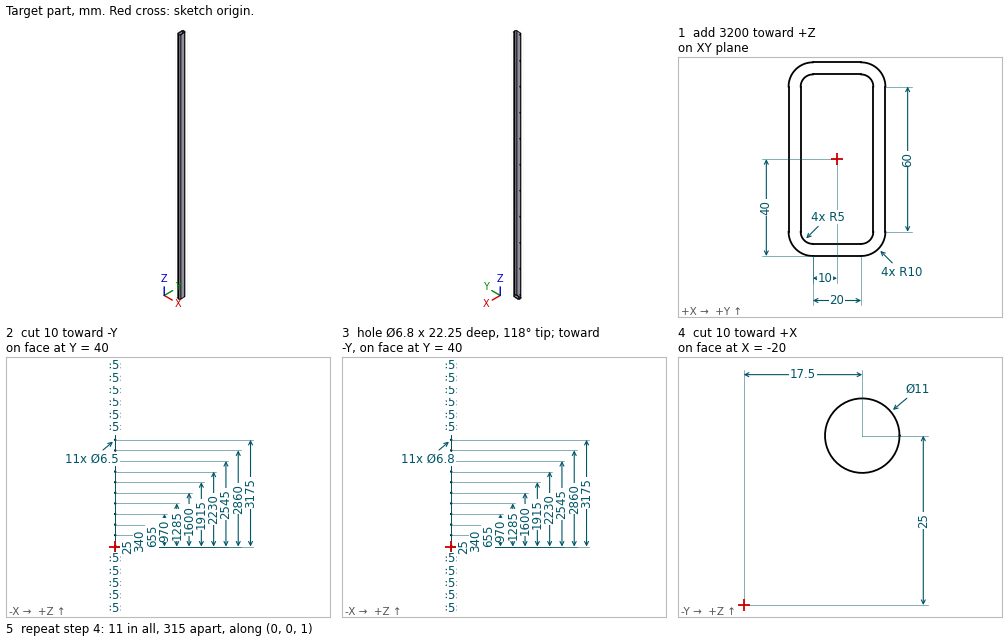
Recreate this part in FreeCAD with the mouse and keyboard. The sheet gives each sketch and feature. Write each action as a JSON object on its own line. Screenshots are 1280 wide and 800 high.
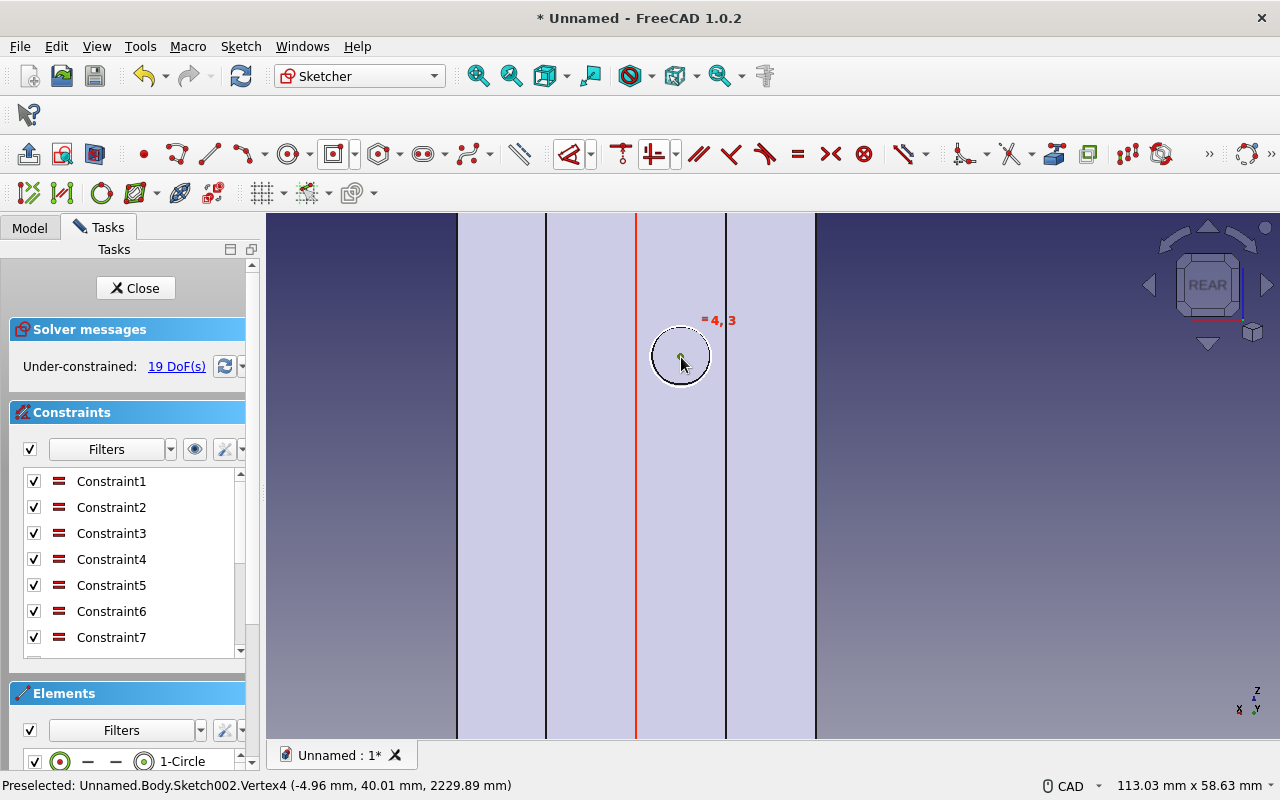
{"action": "left_click", "coordinate": [590, 154]}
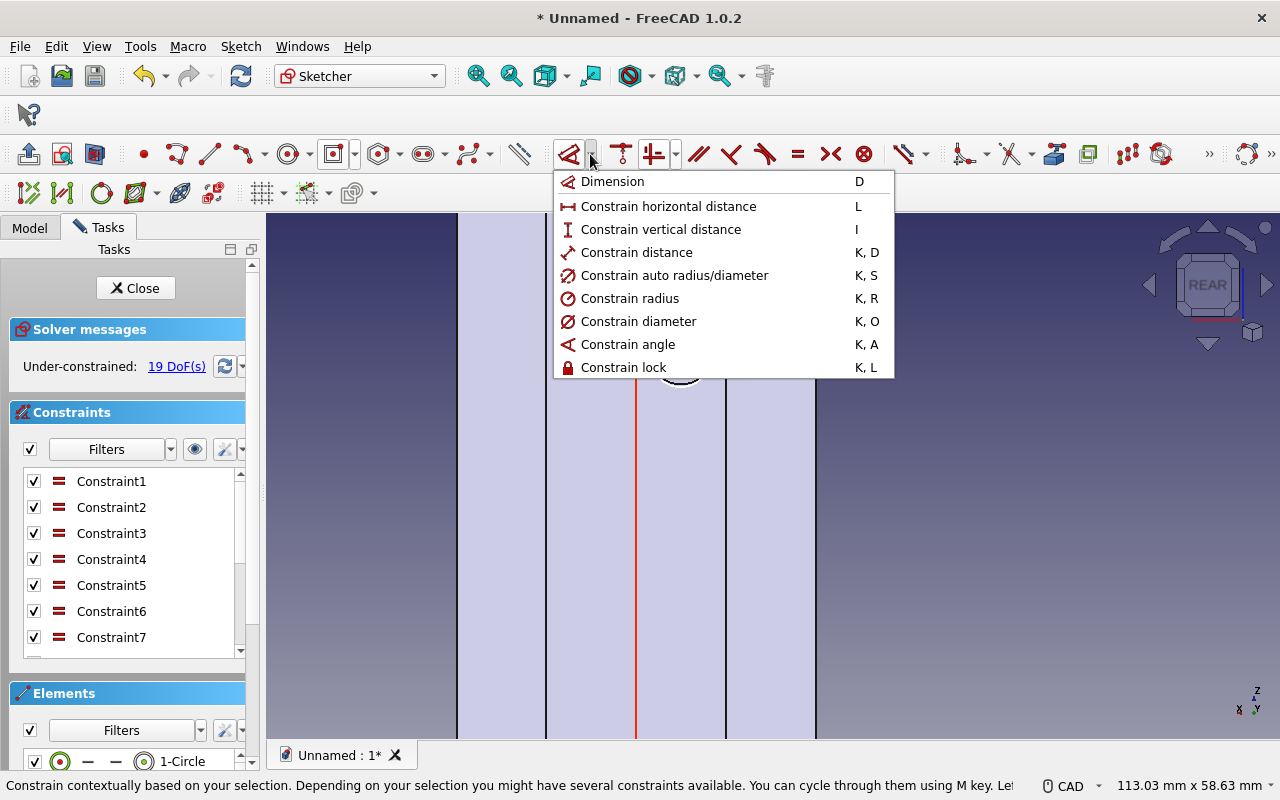
{"action": "left_click", "coordinate": [724, 206]}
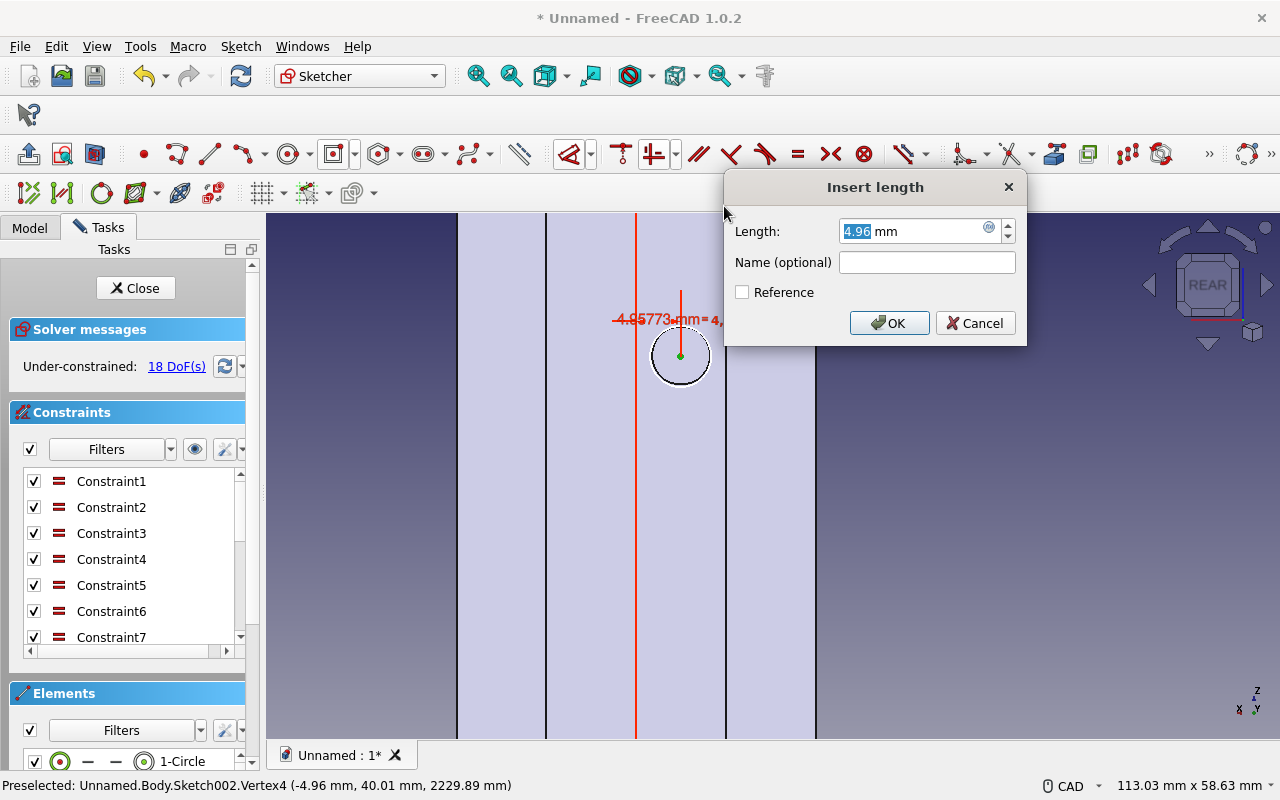
{"action": "type", "text": "5"}
{"action": "key", "text": "Return"}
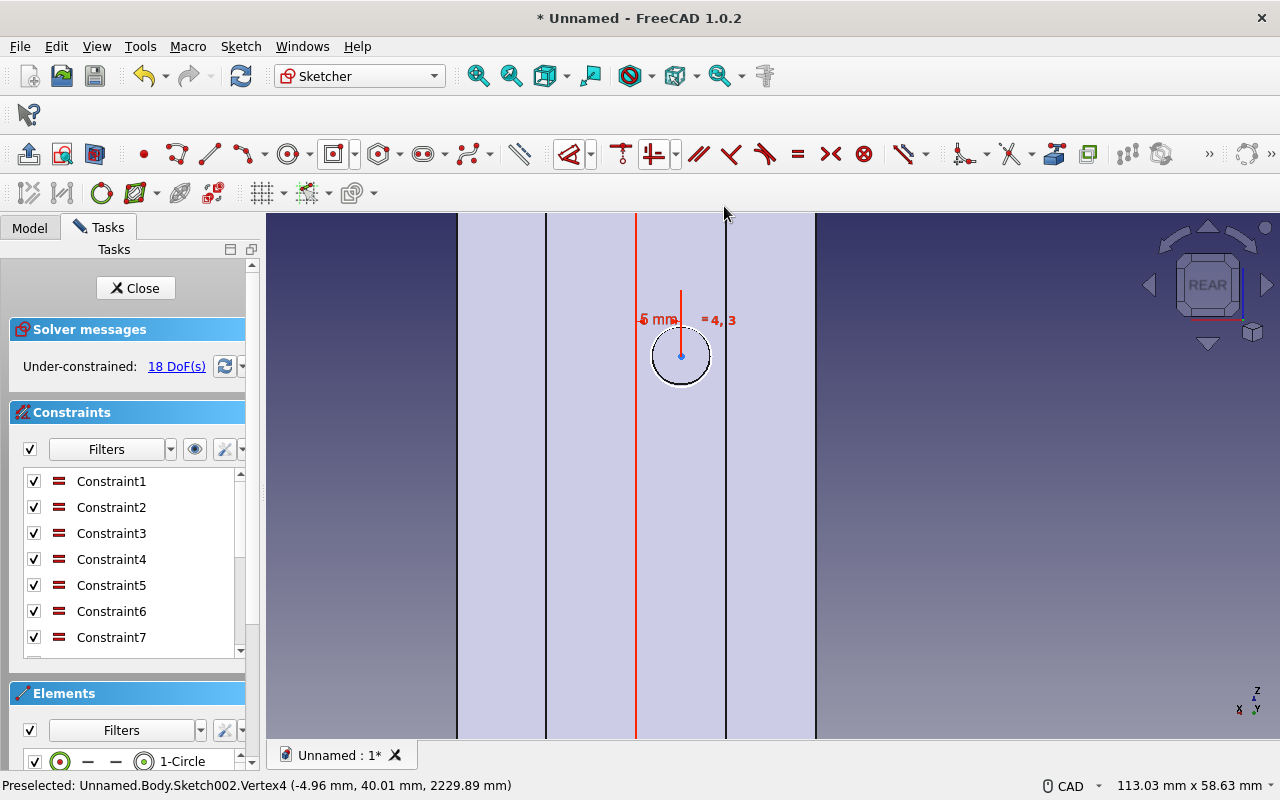
{"action": "scroll", "coordinate": [704, 476], "scroll_direction": "down", "scroll_amount": 15}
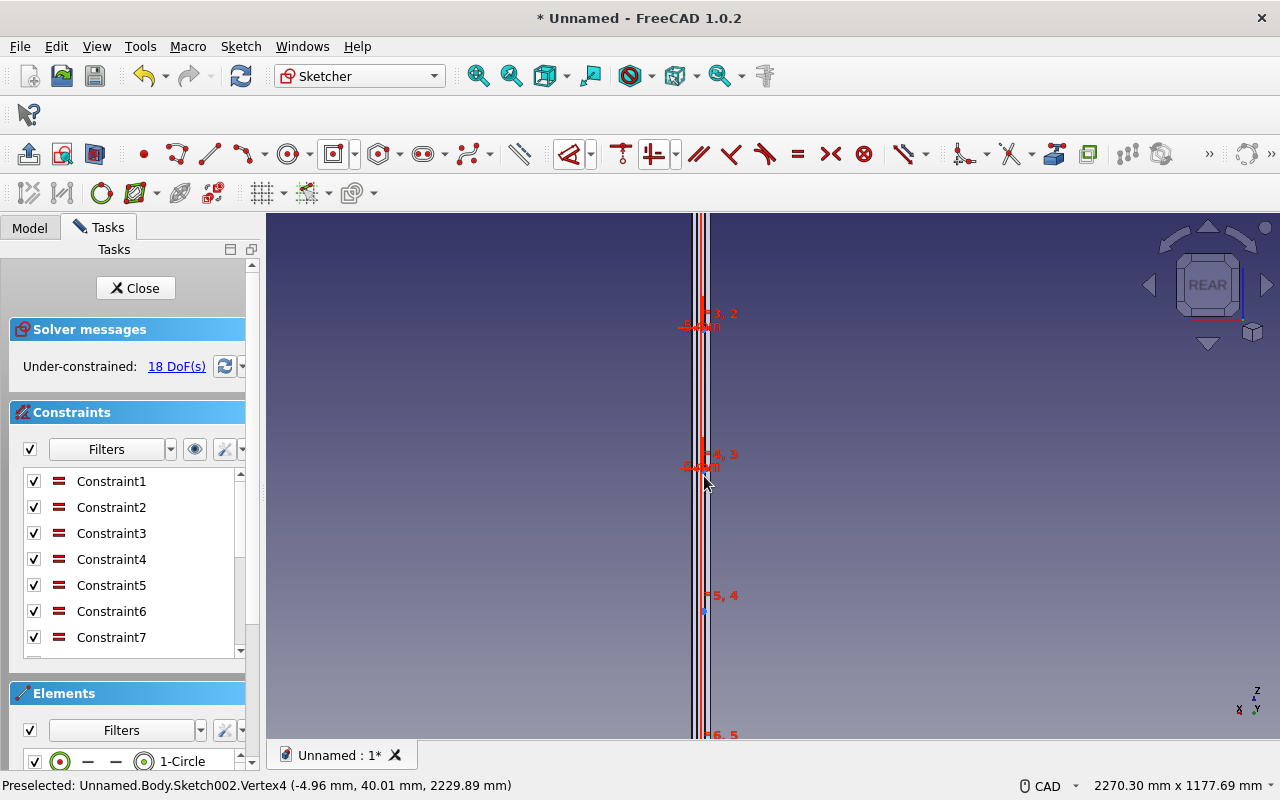
{"action": "scroll", "coordinate": [705, 384], "scroll_direction": "down", "scroll_amount": 7}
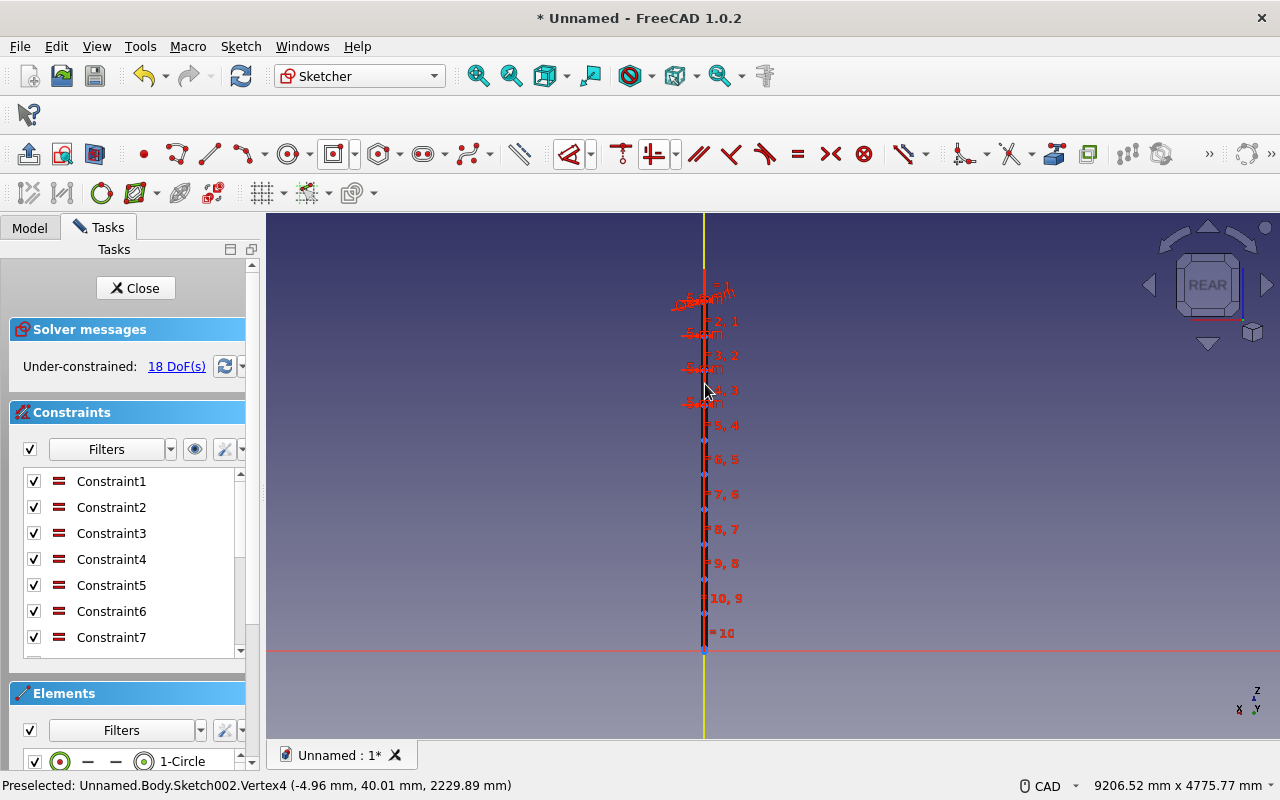
{"action": "scroll", "coordinate": [705, 440], "scroll_direction": "up", "scroll_amount": 22}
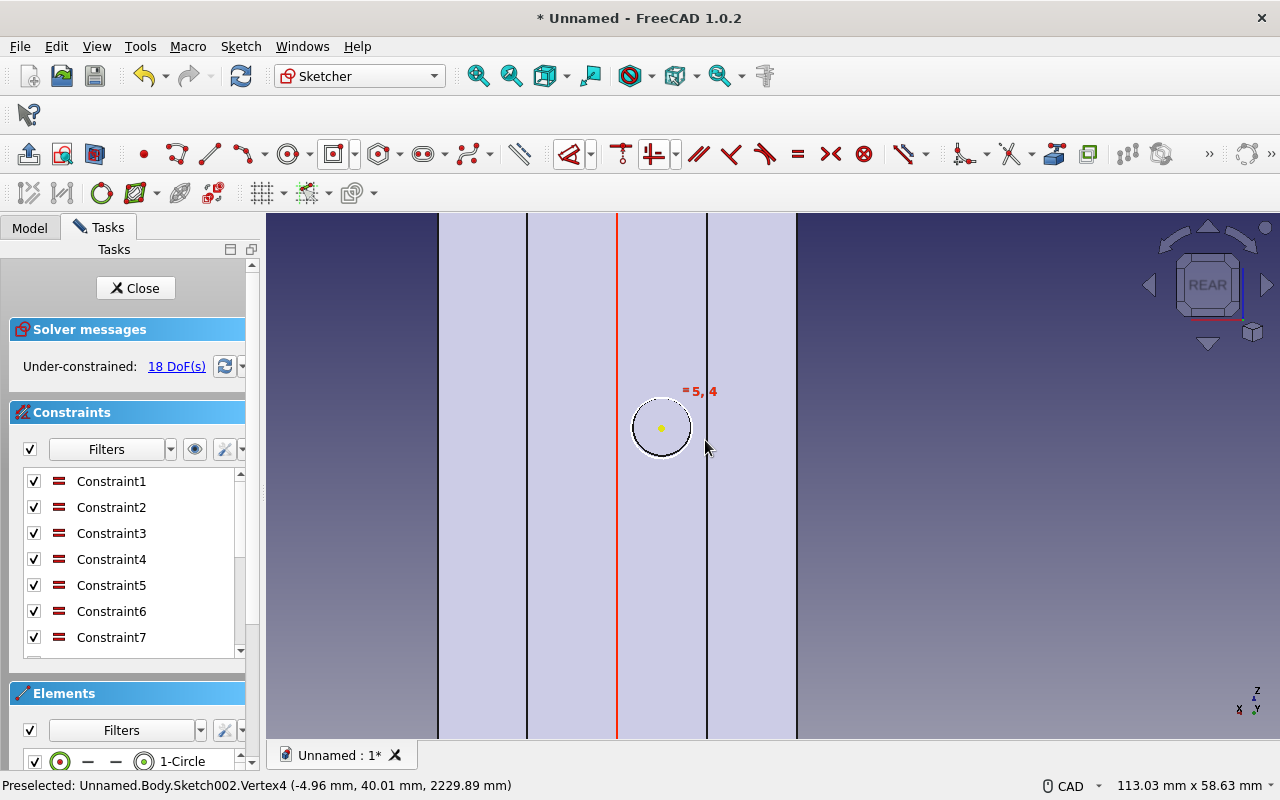
{"action": "left_click", "coordinate": [662, 428]}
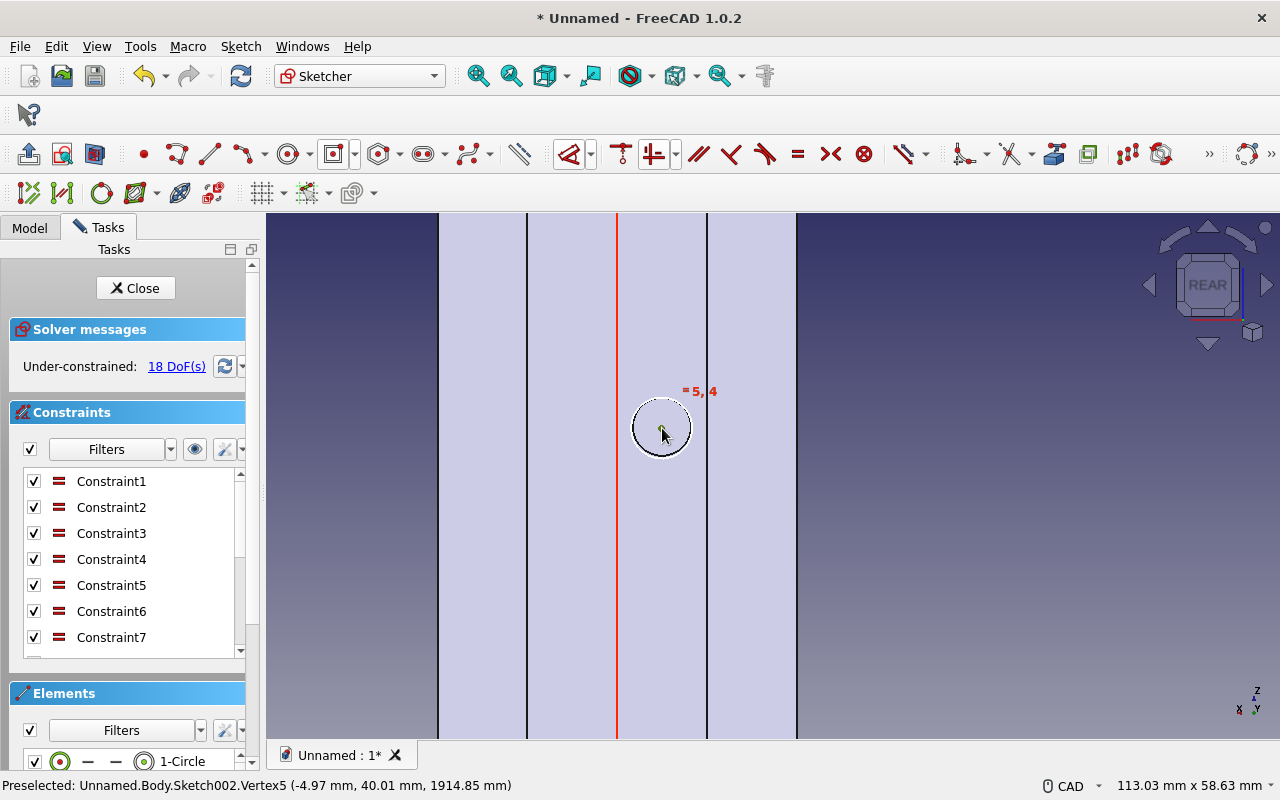
{"action": "key", "text": "l"}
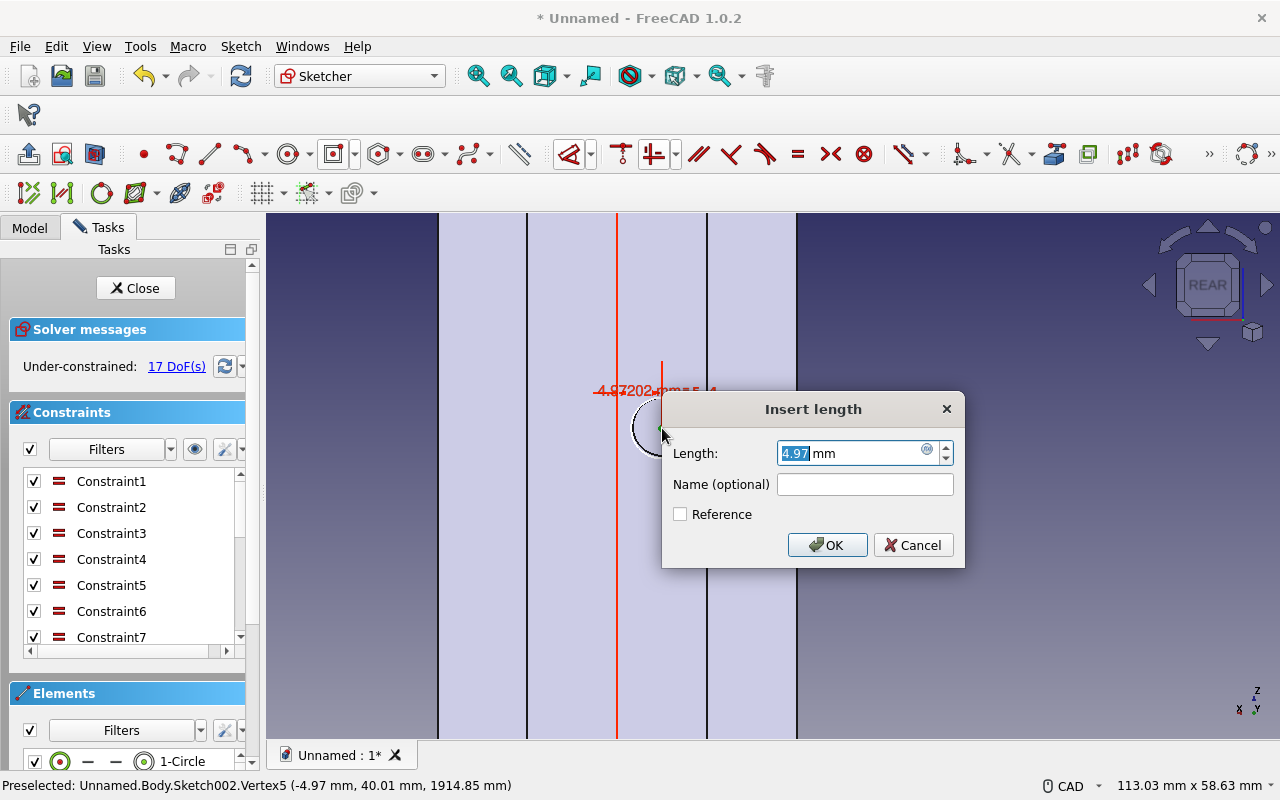
{"action": "type", "text": "5"}
{"action": "key", "text": "Return"}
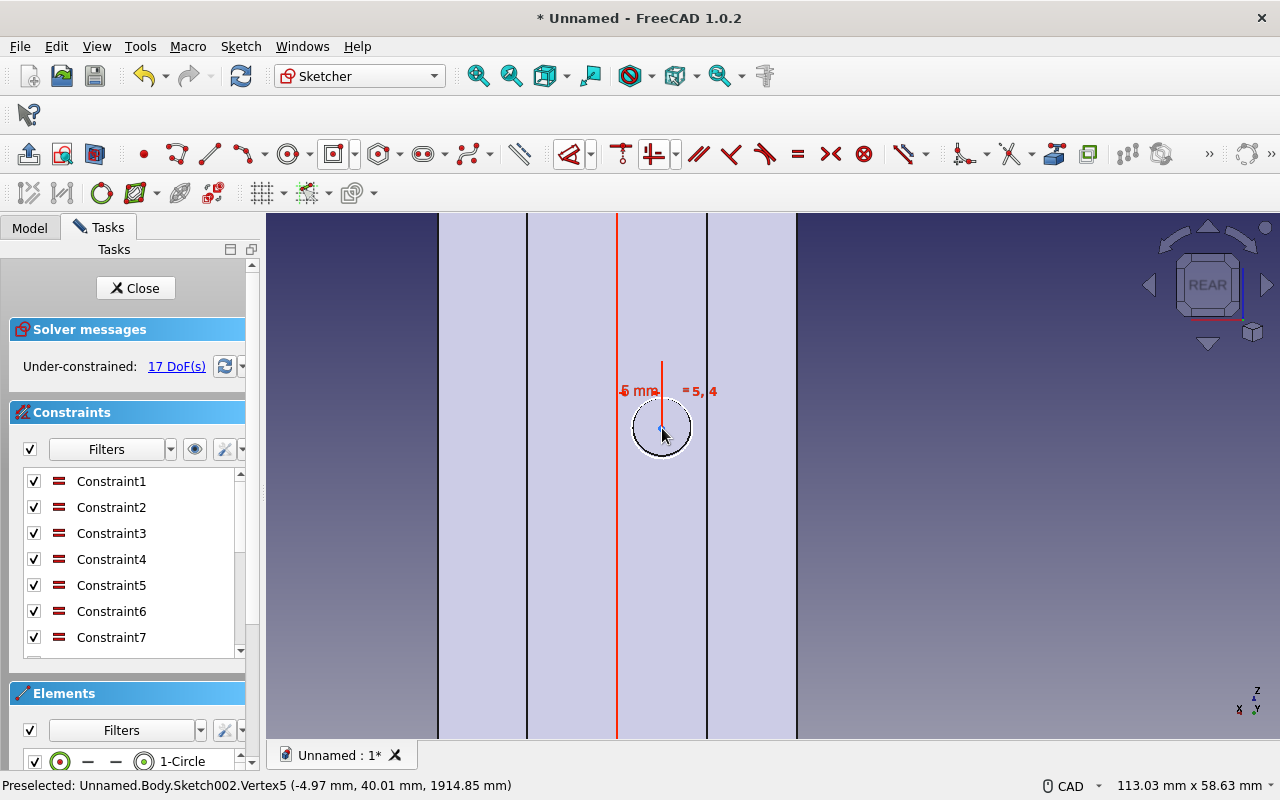
{"action": "scroll", "coordinate": [704, 476], "scroll_direction": "down", "scroll_amount": 15}